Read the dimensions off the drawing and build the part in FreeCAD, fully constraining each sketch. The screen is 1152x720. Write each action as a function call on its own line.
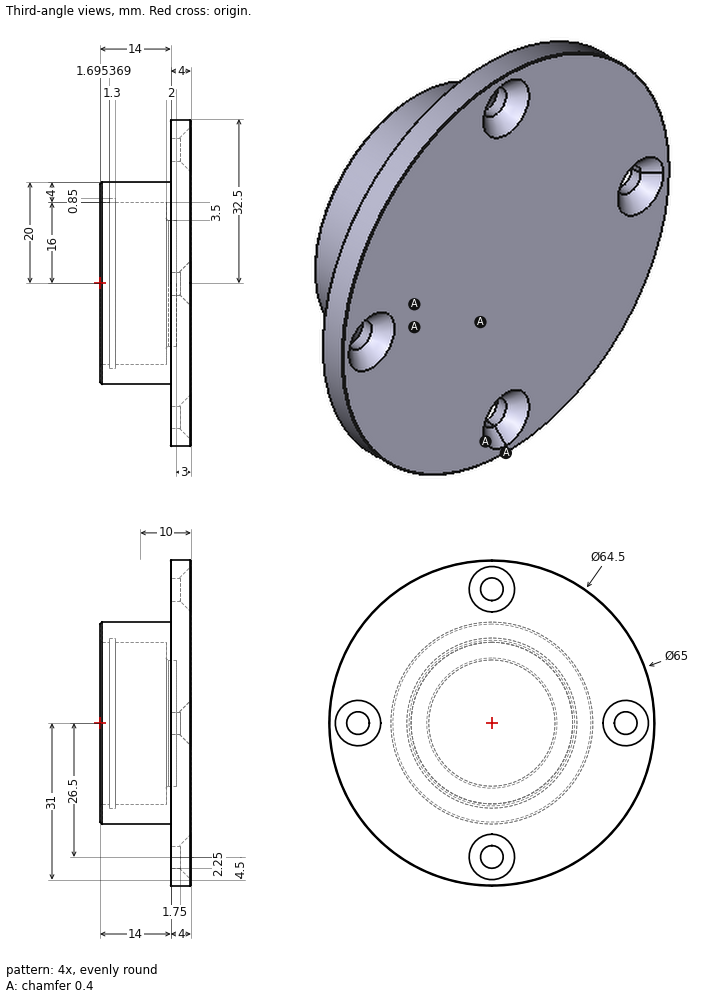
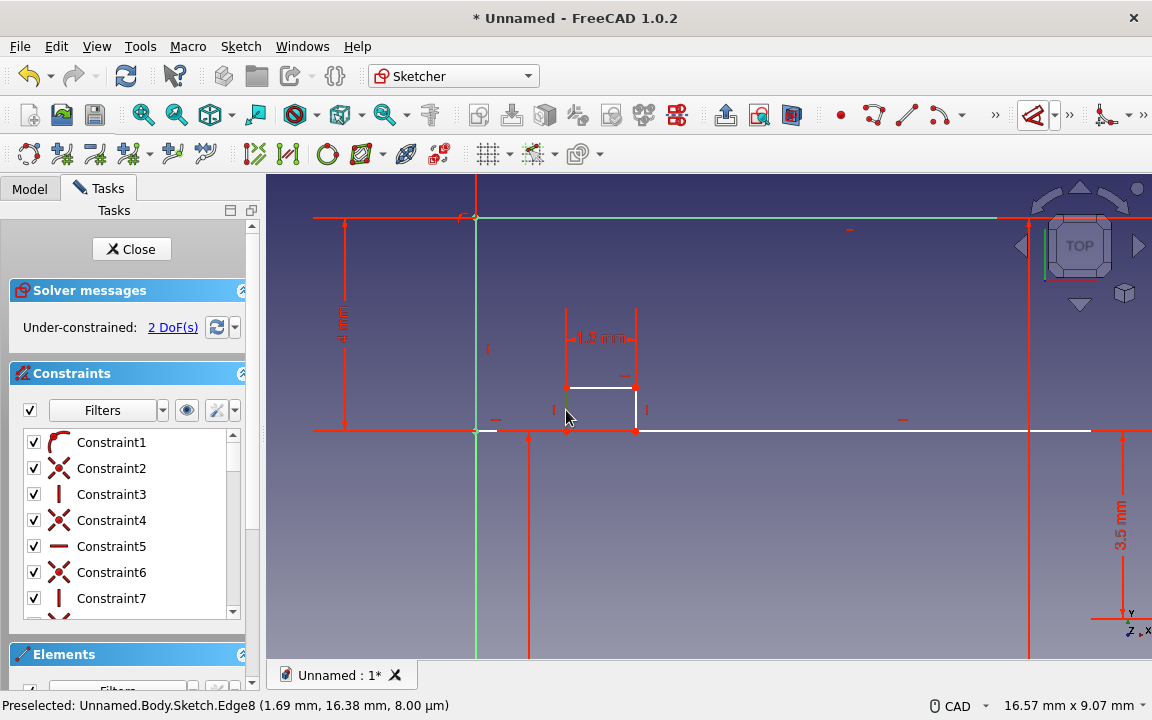
click(1054, 116)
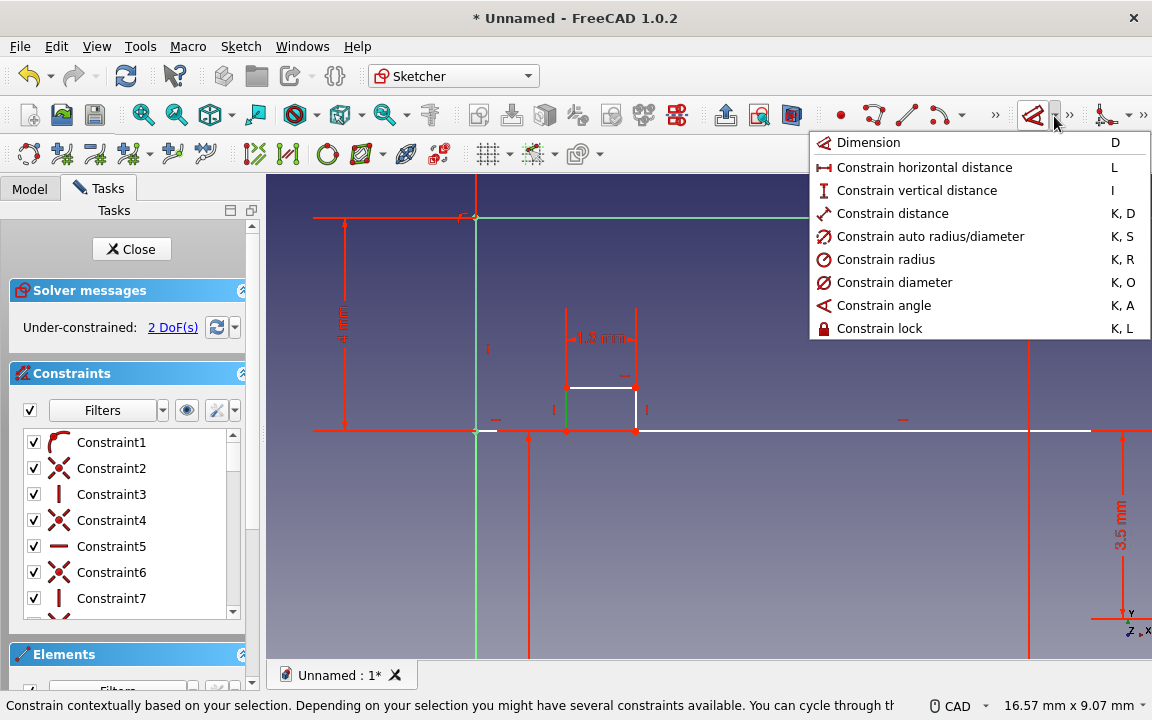
click(980, 190)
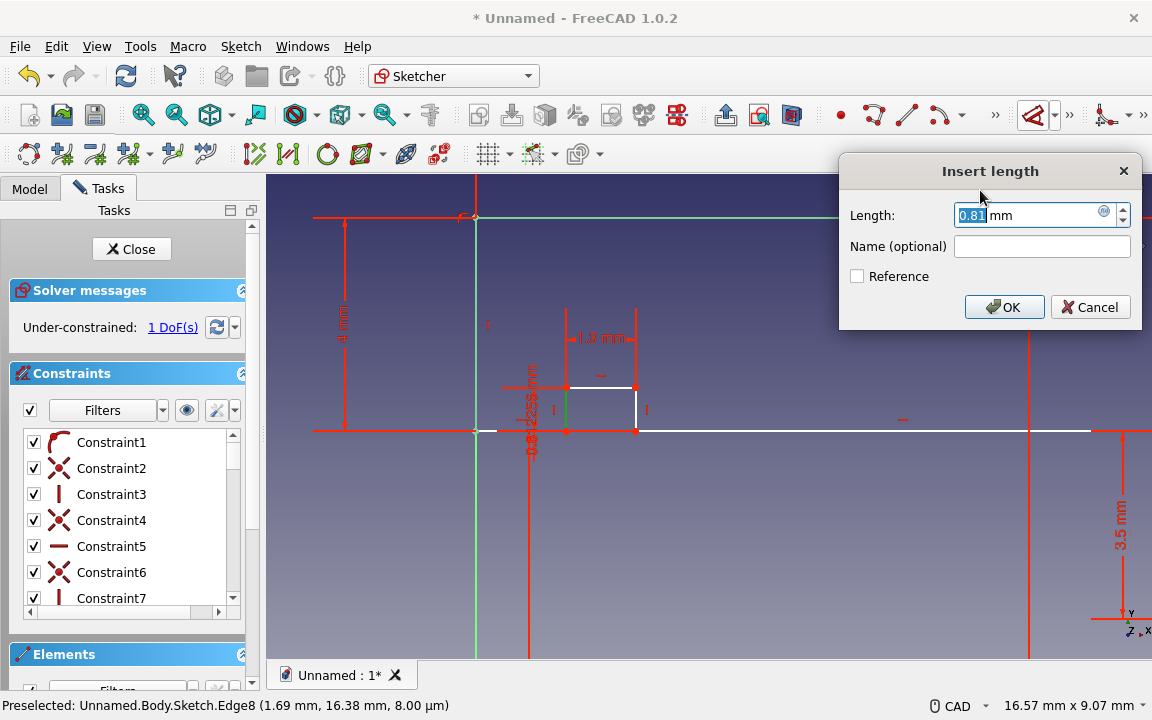
text(0.85)
key(Return)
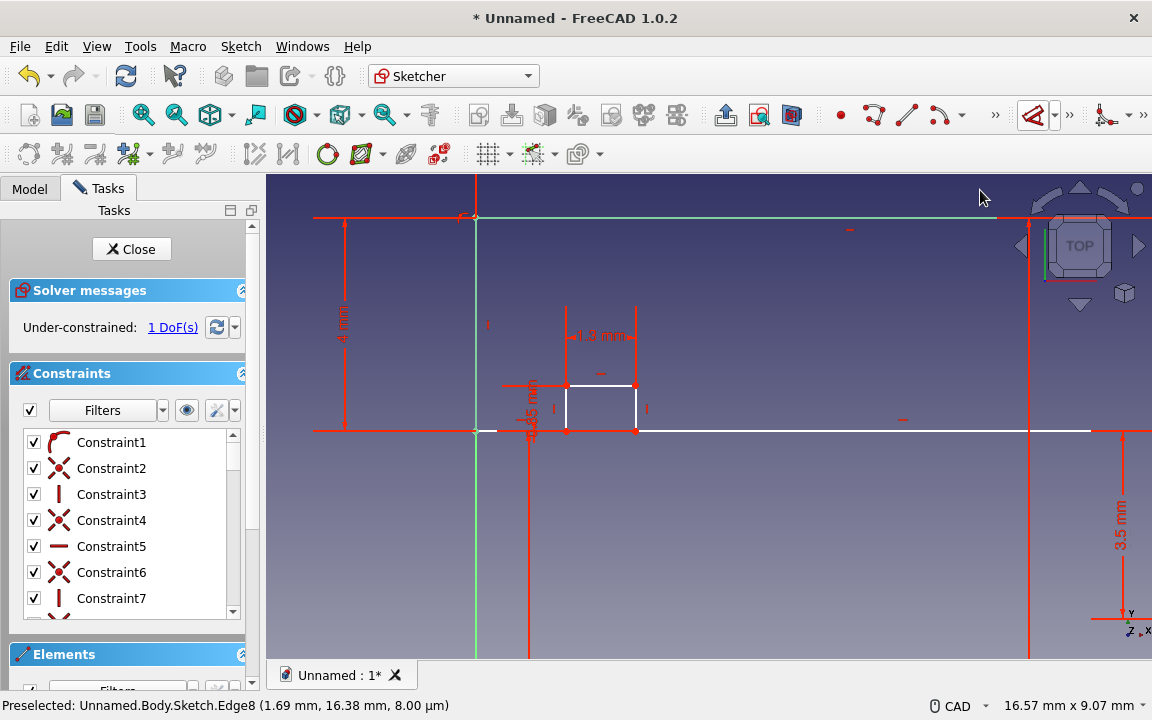
click(503, 431)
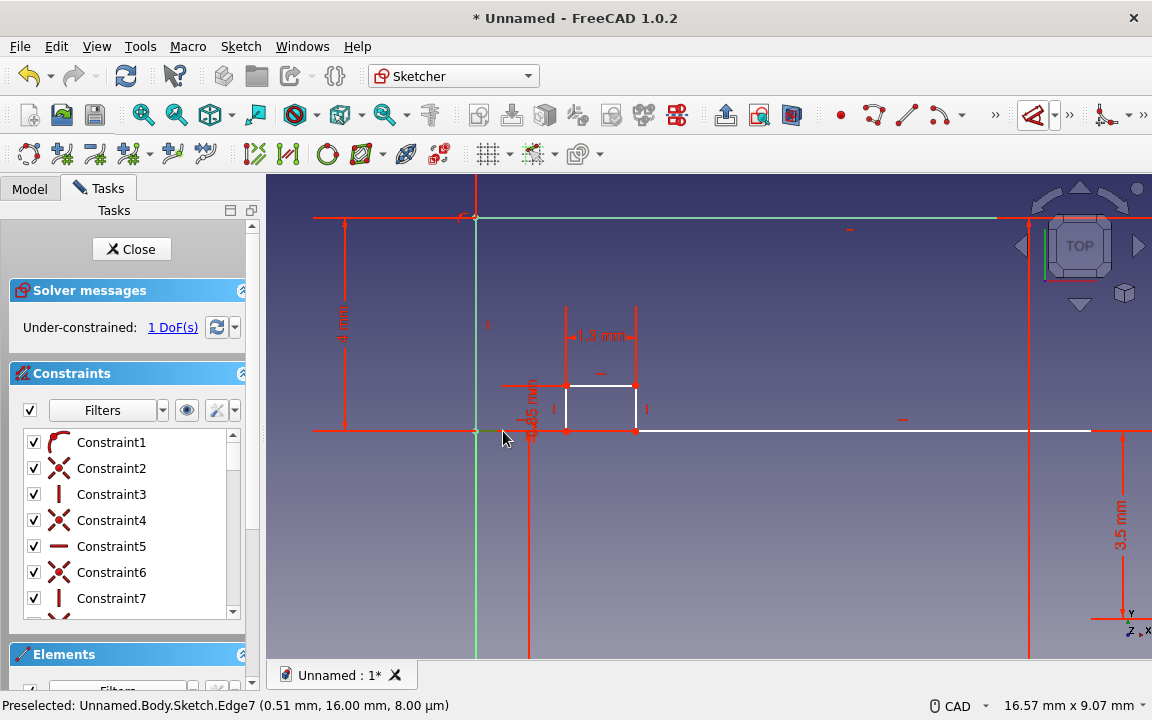
click(1054, 116)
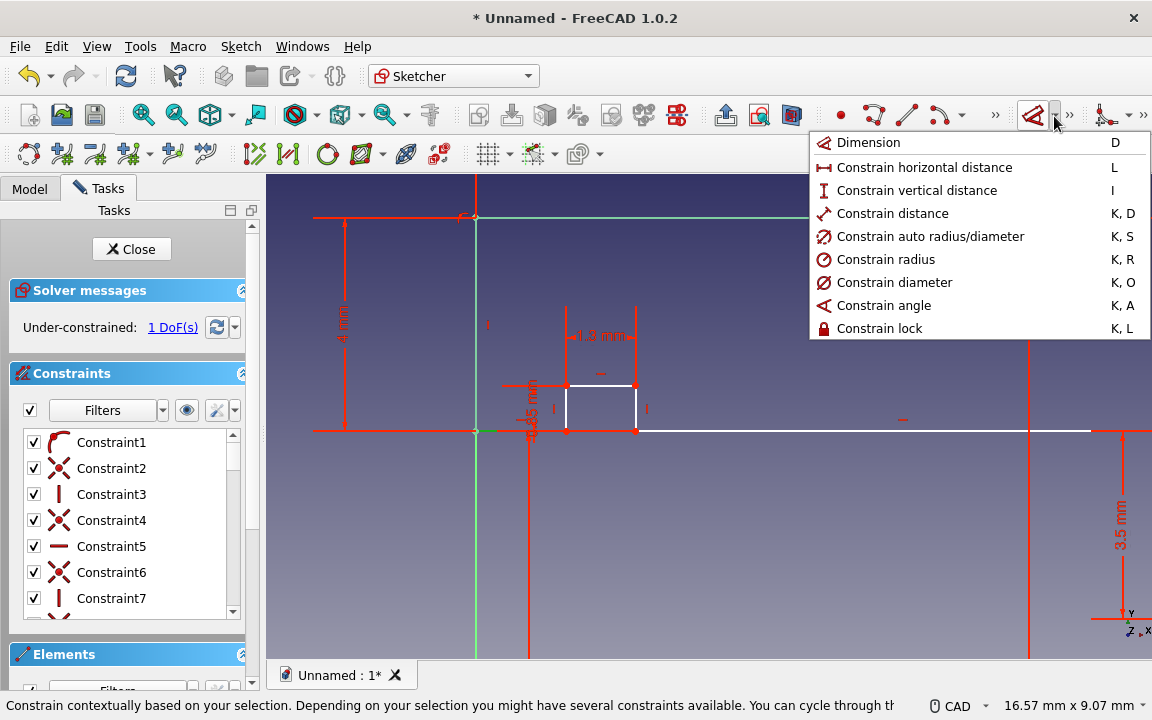
click(980, 168)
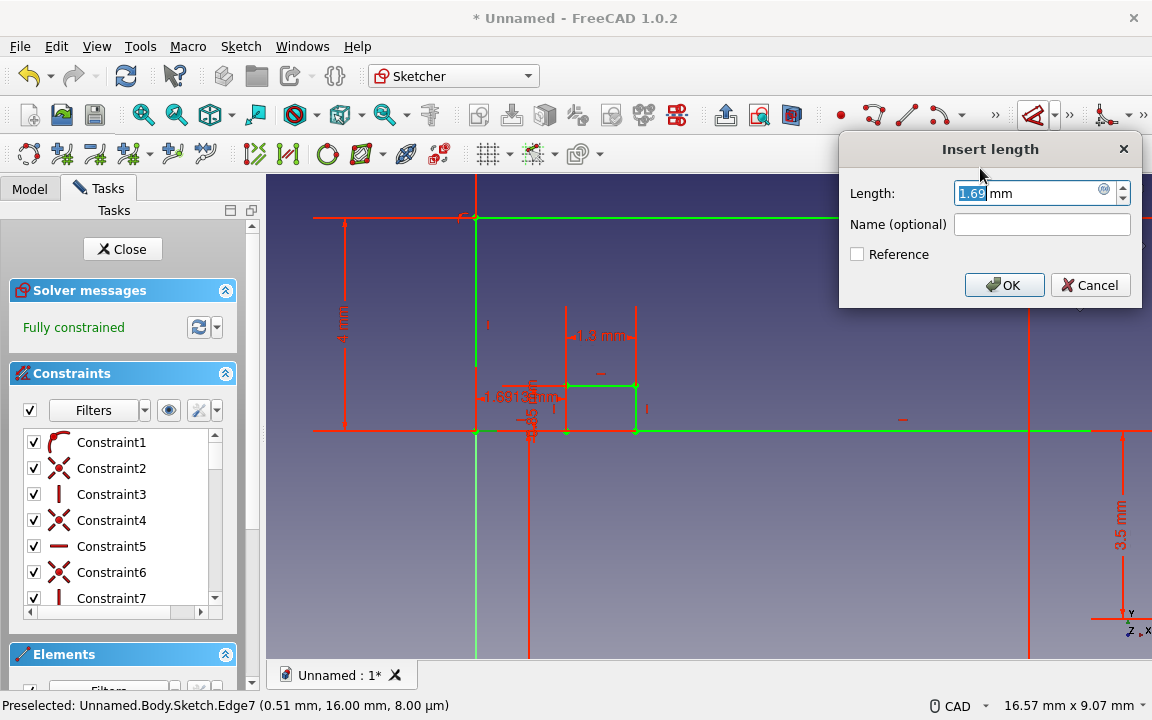
text(1.695369)
key(Return)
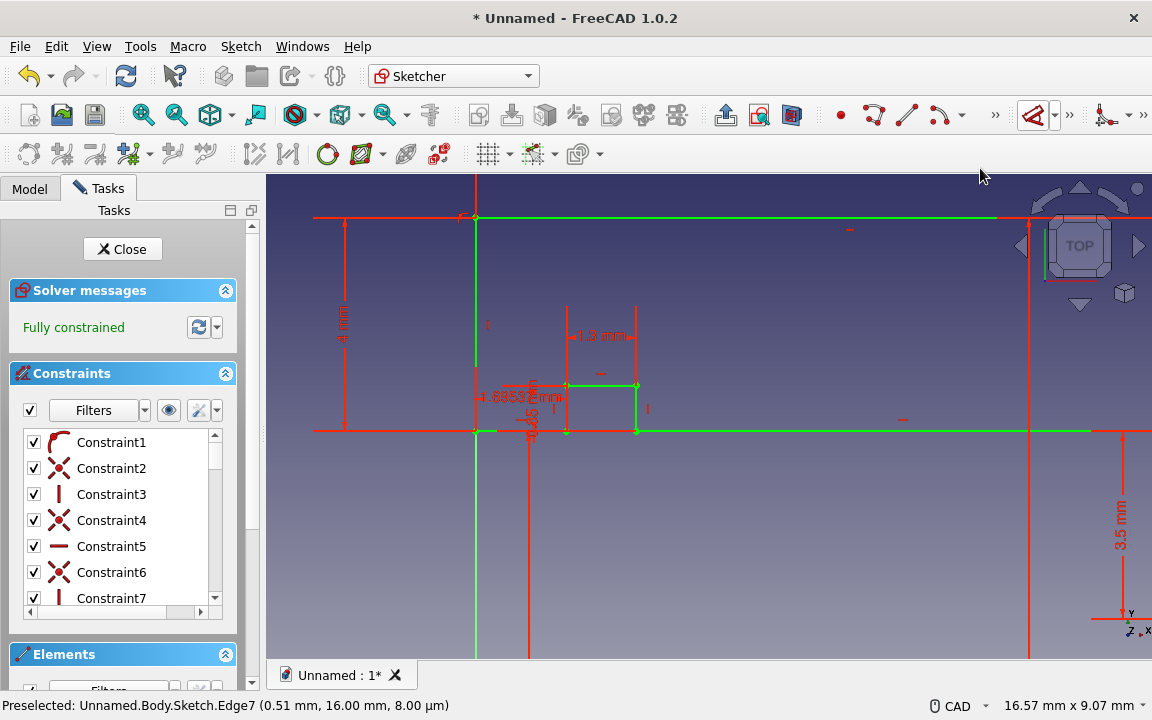
click(123, 249)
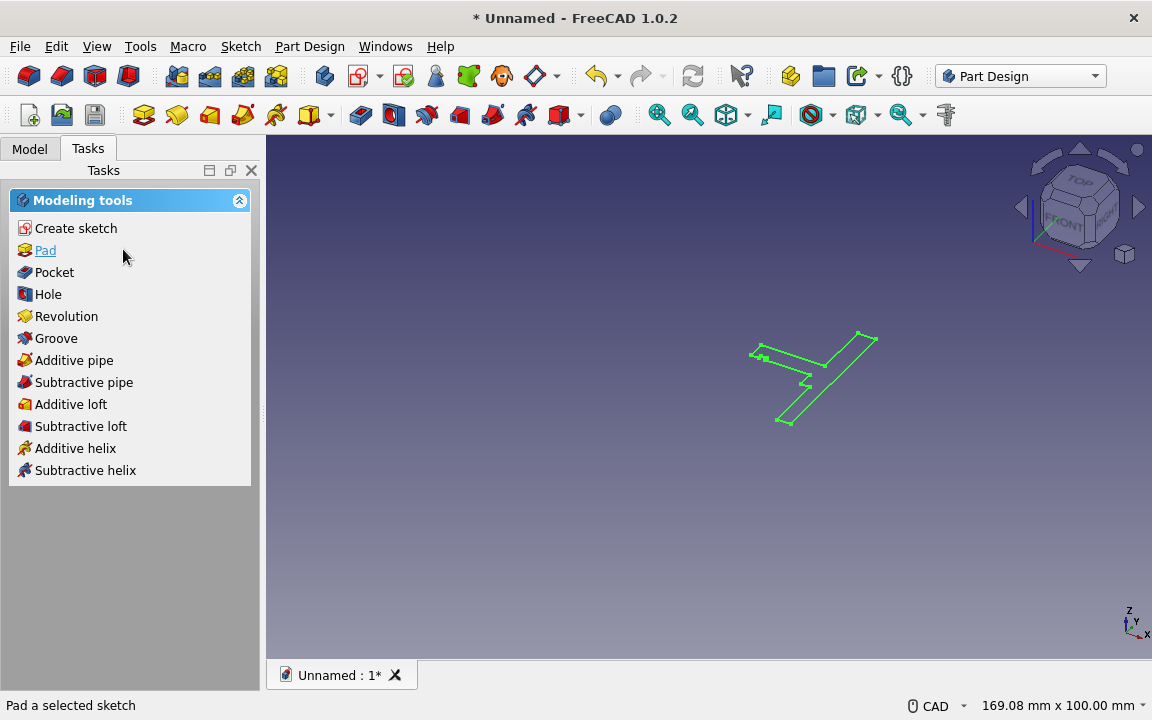
click(177, 116)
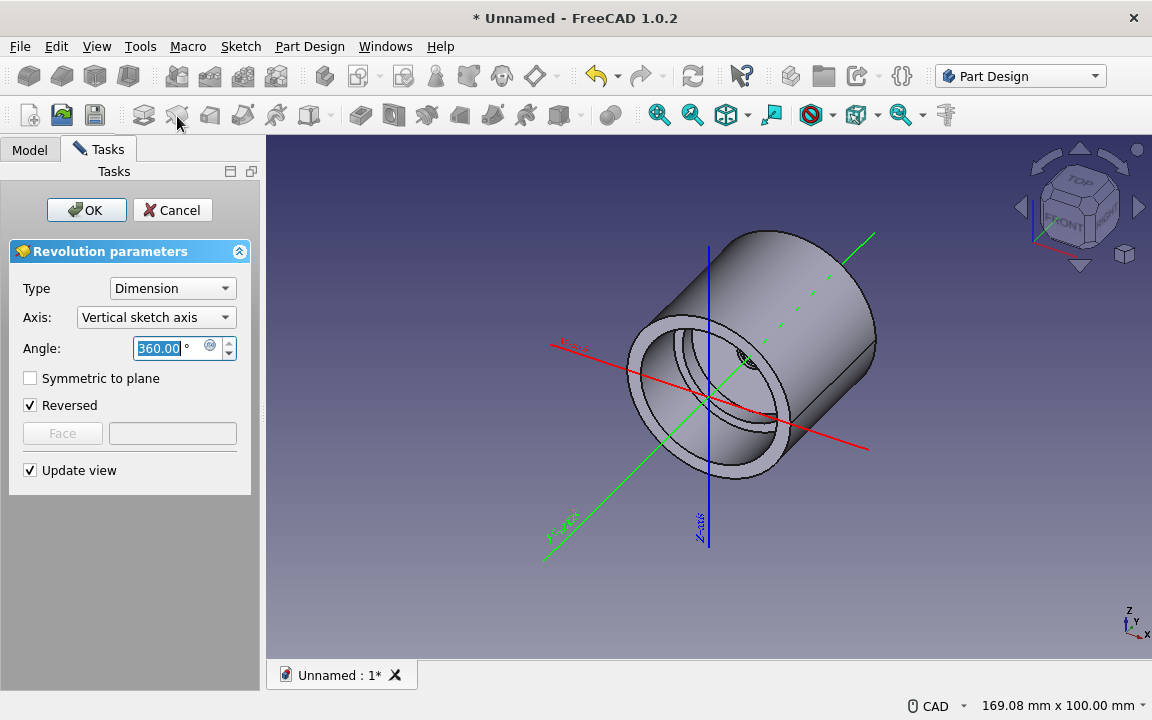
click(157, 318)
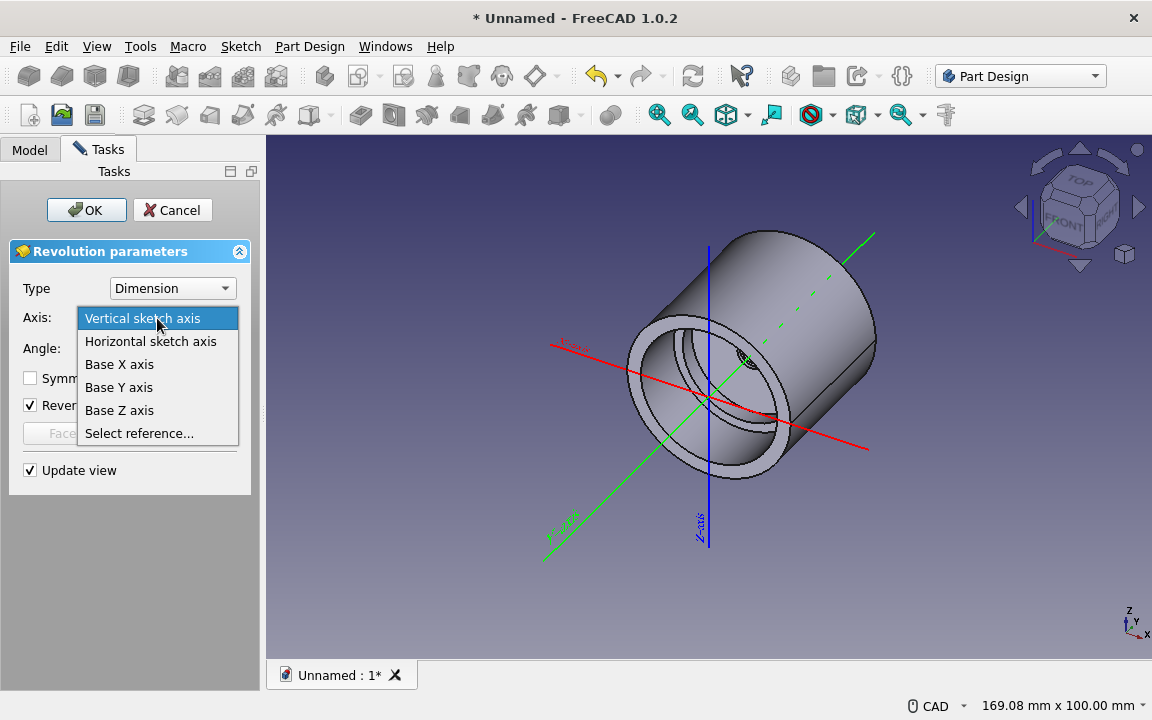
click(156, 342)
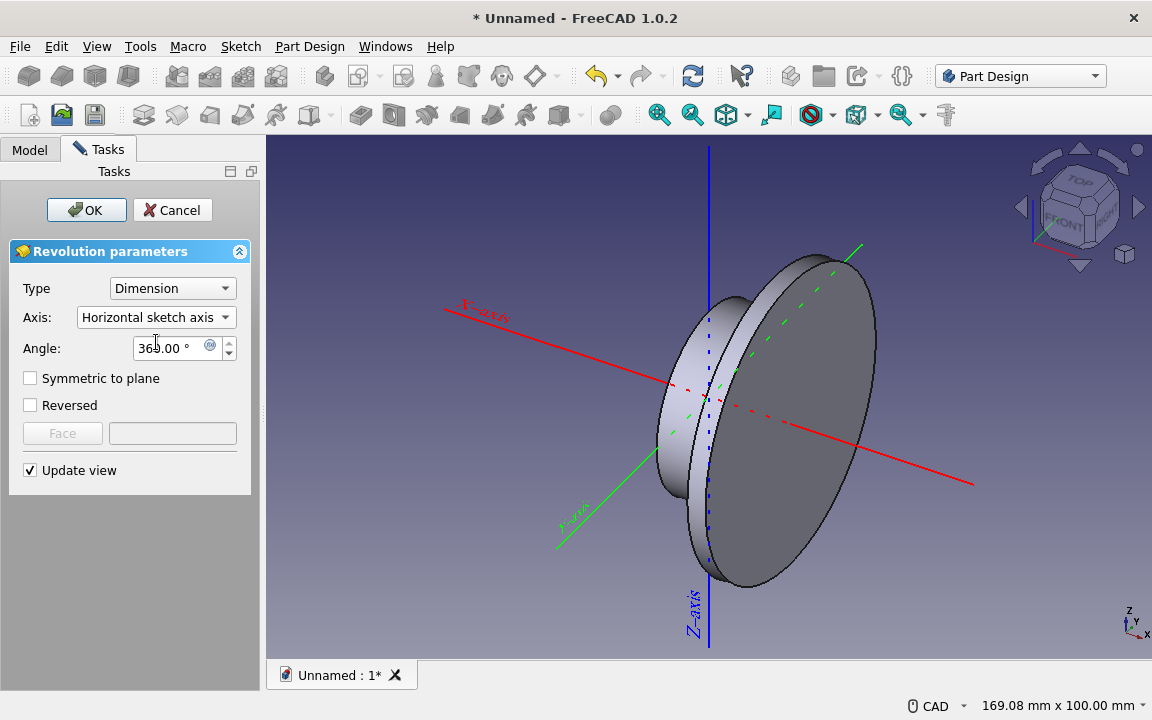
click(87, 210)